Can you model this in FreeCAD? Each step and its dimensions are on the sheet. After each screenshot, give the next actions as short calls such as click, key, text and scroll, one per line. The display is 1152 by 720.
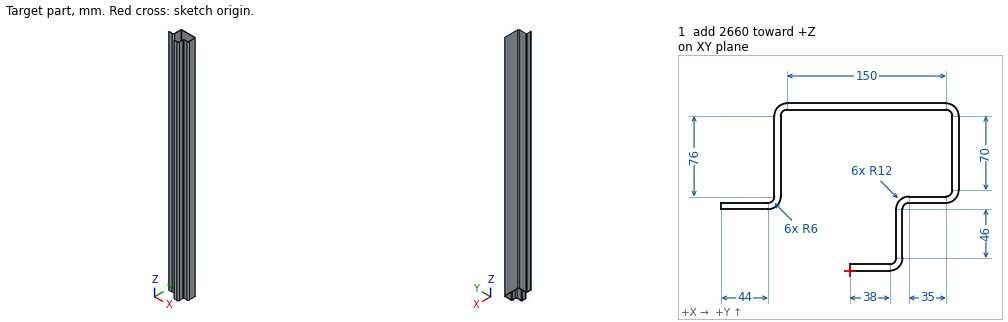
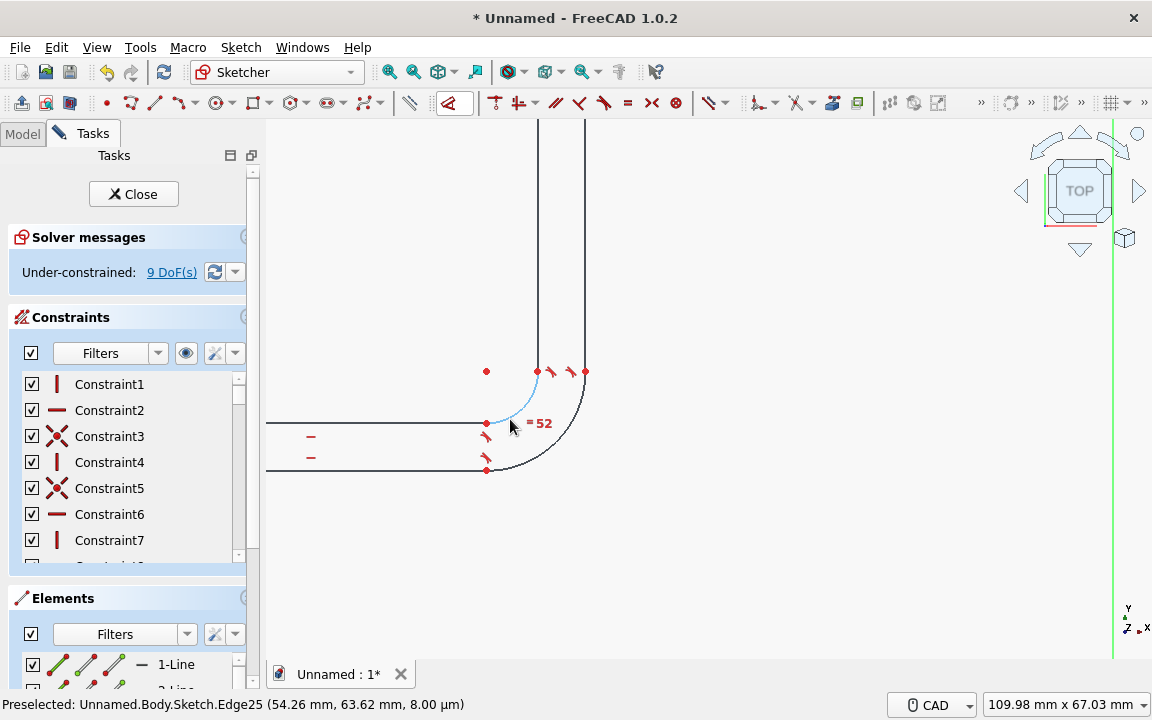
click(510, 418)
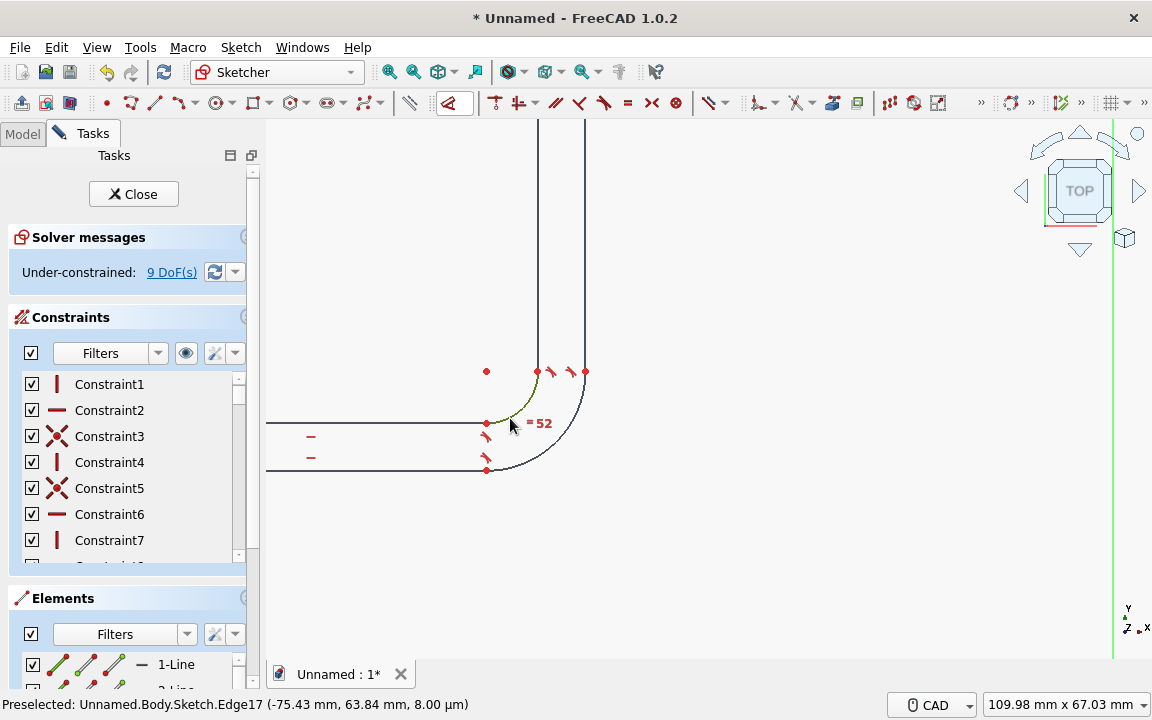
key(k)
key(r)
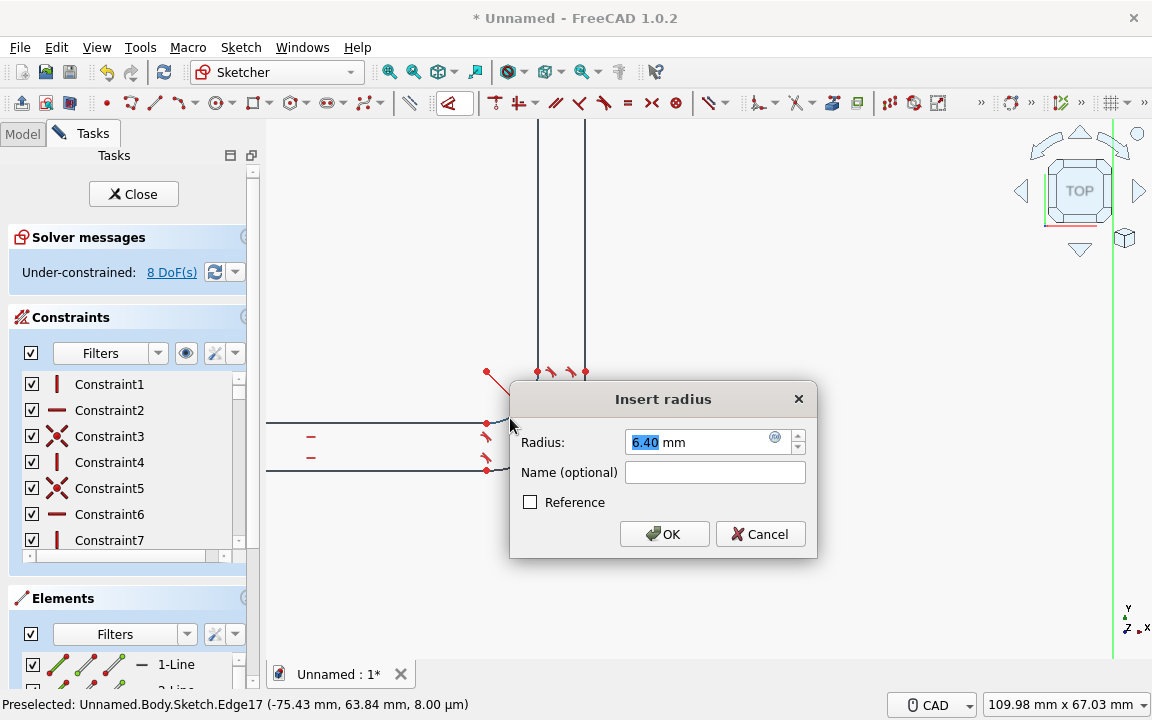
text(6)
key(Return)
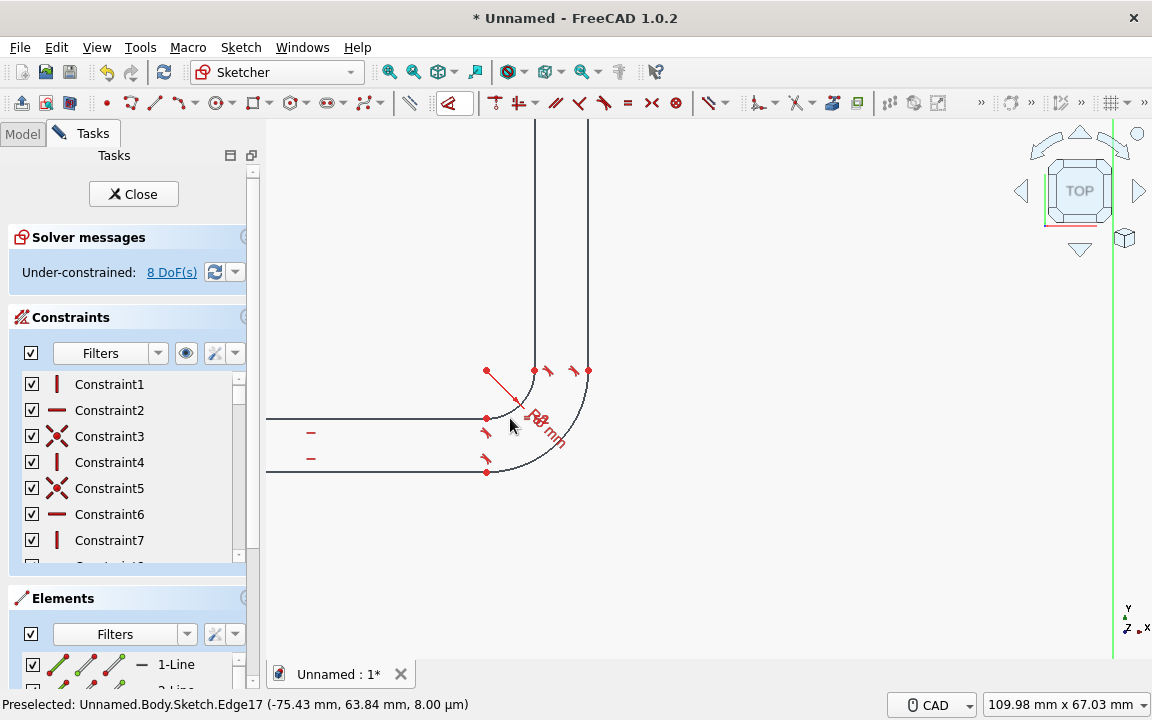
click(533, 461)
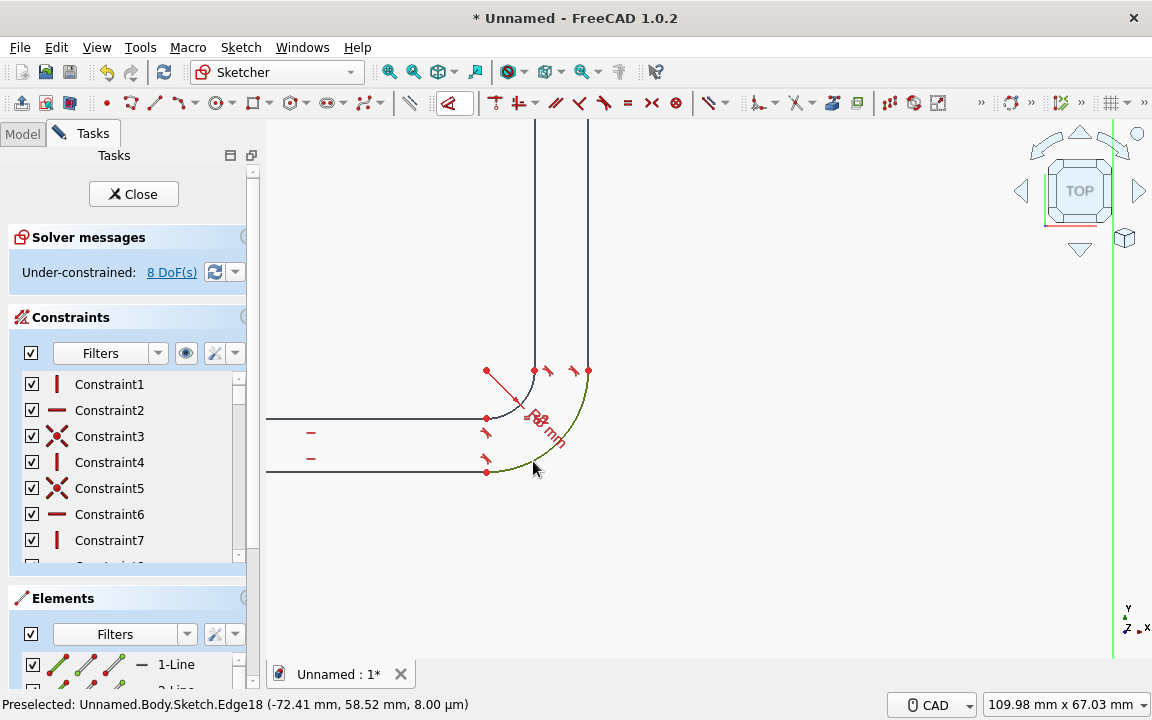
click(468, 104)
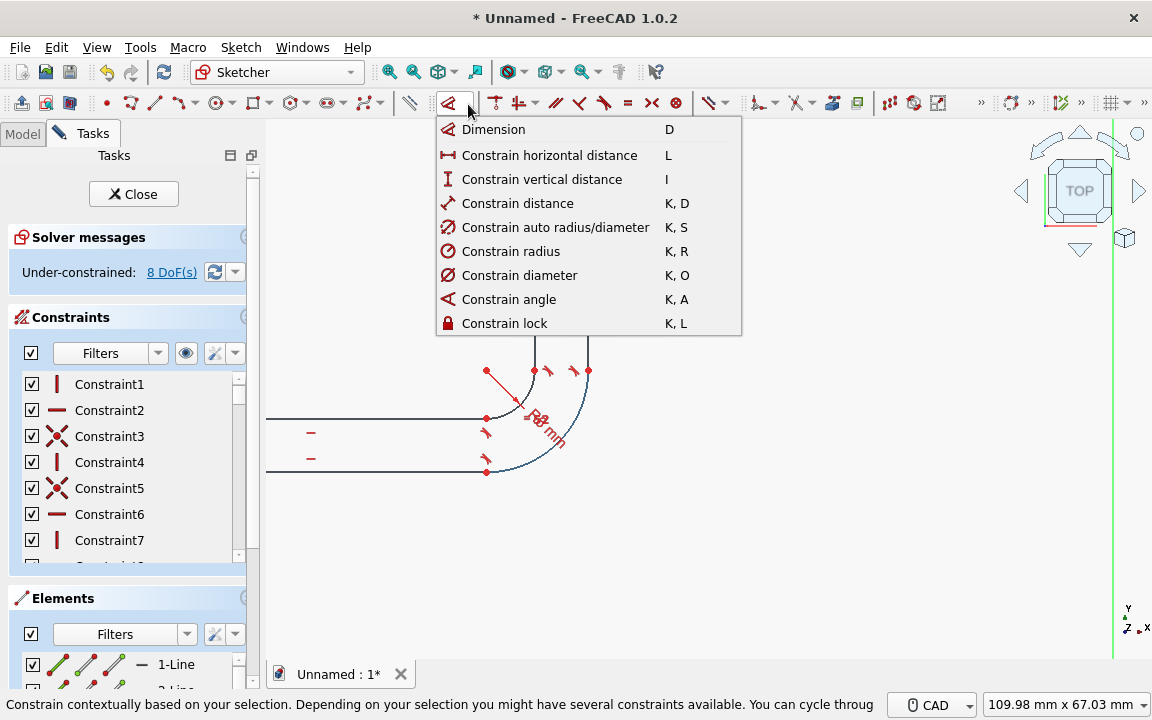
click(589, 251)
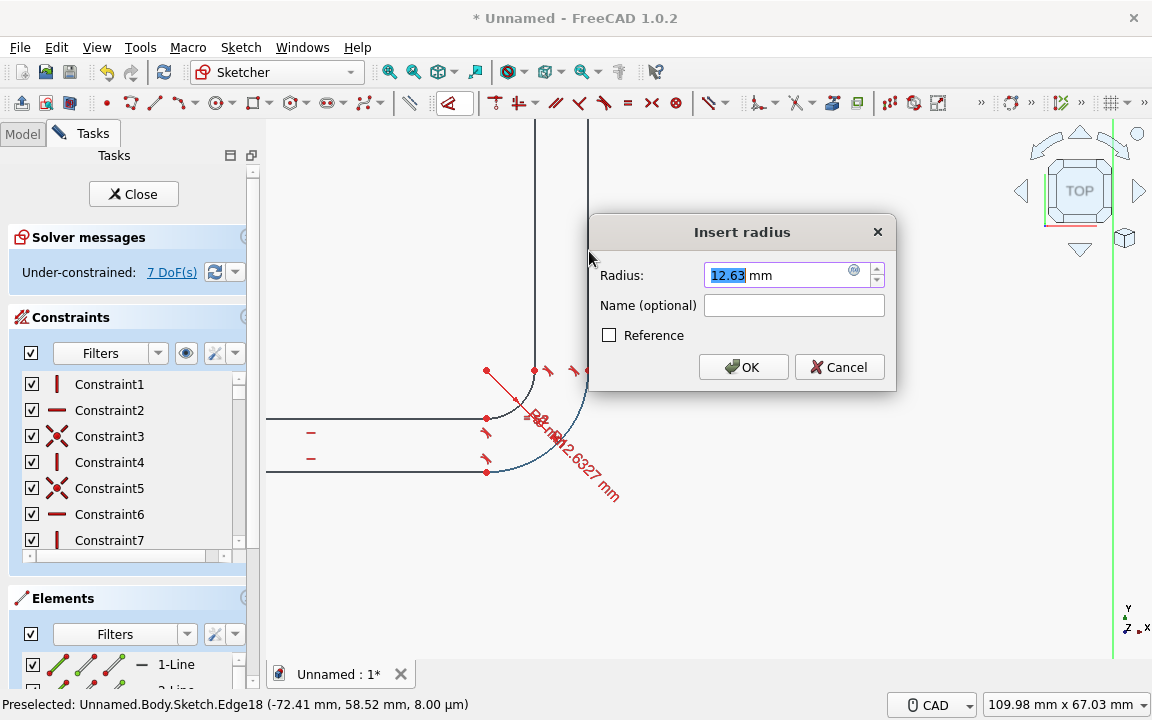
text(12)
key(Return)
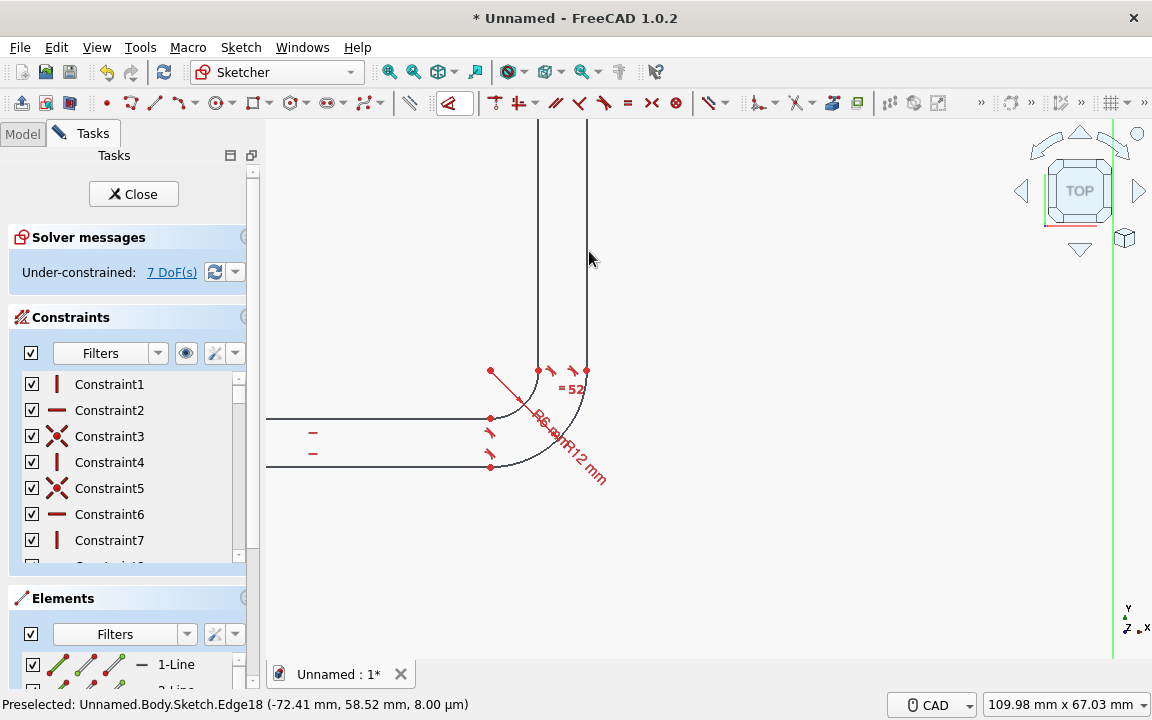
scroll(510, 419, down, 7)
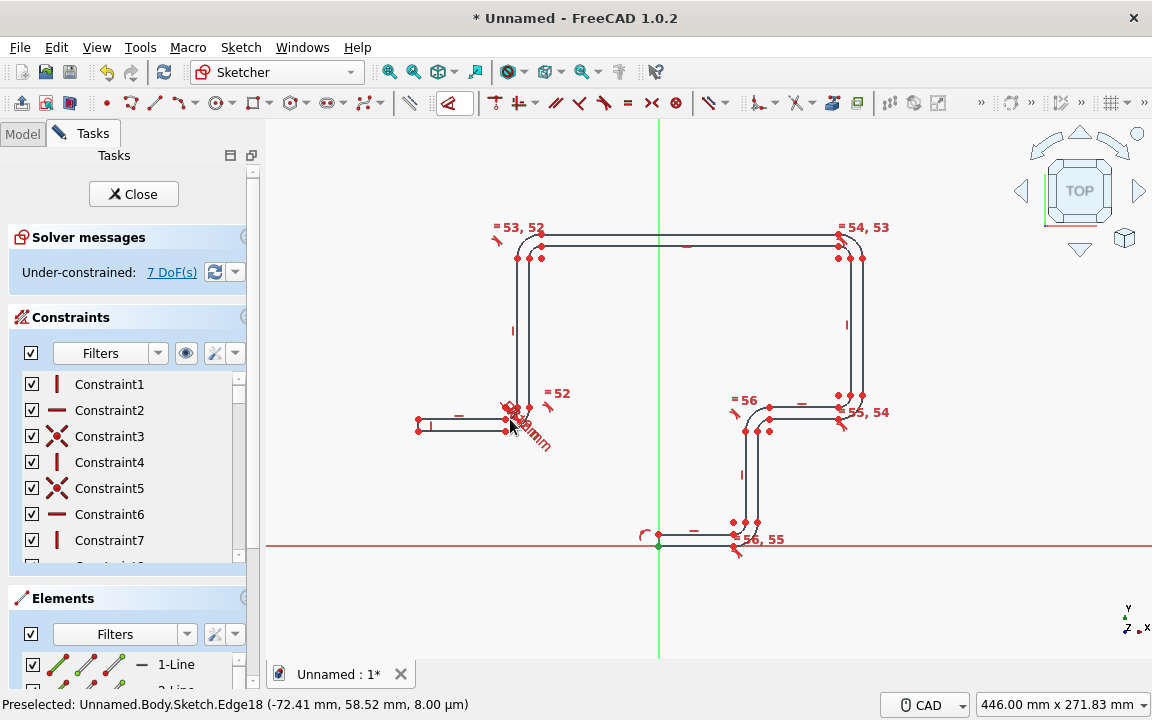
click(517, 363)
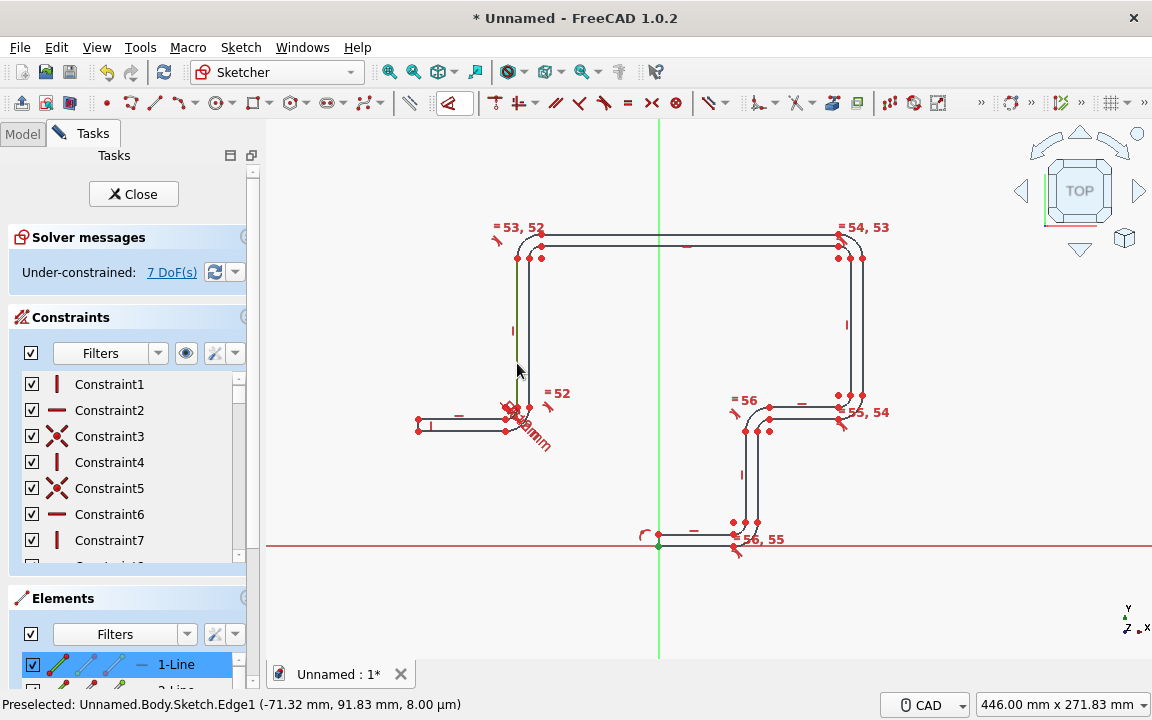
key(i)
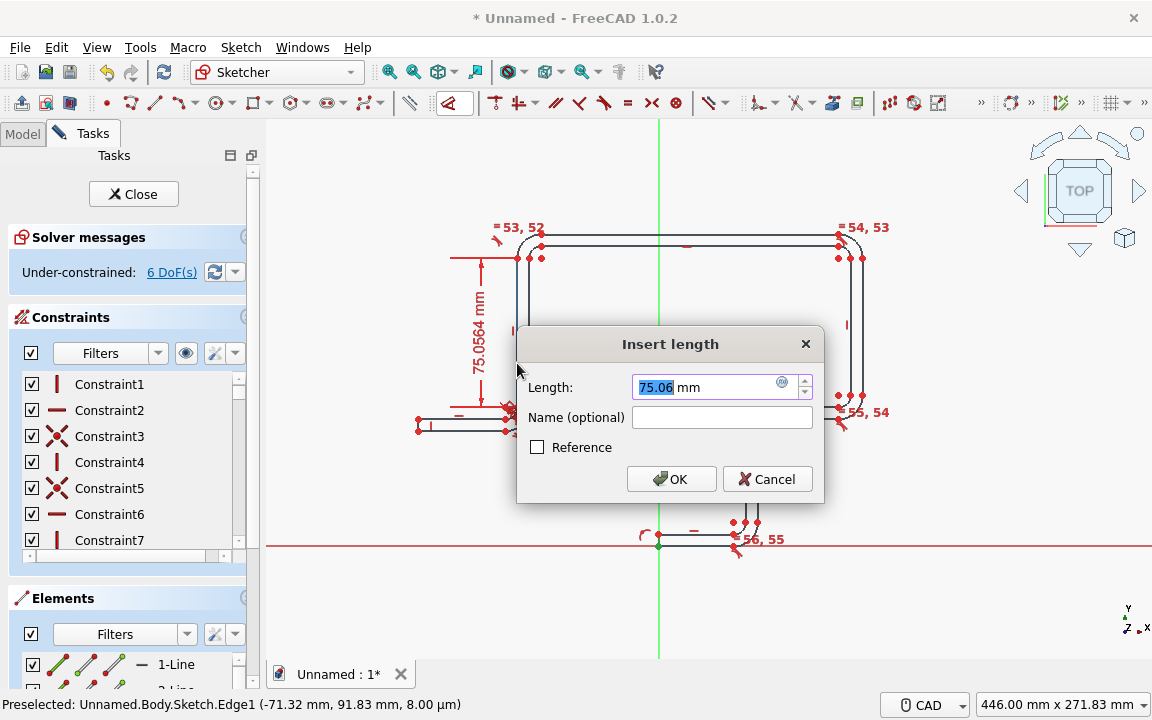
text(76)
key(Return)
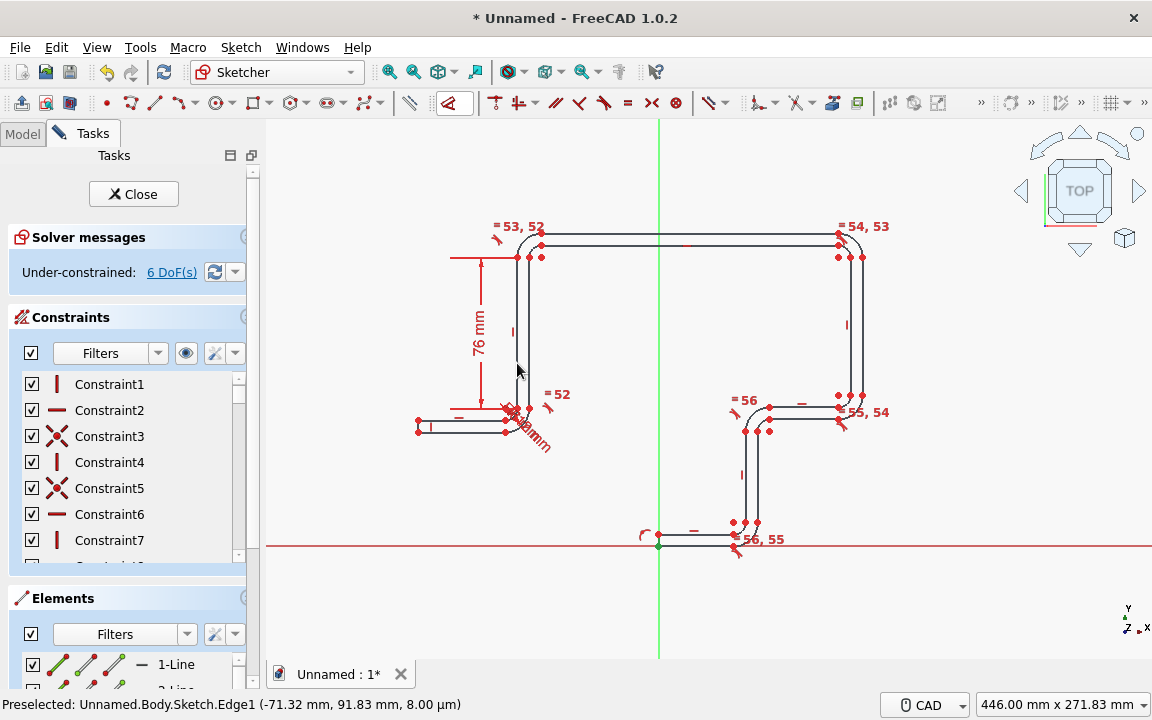
click(479, 421)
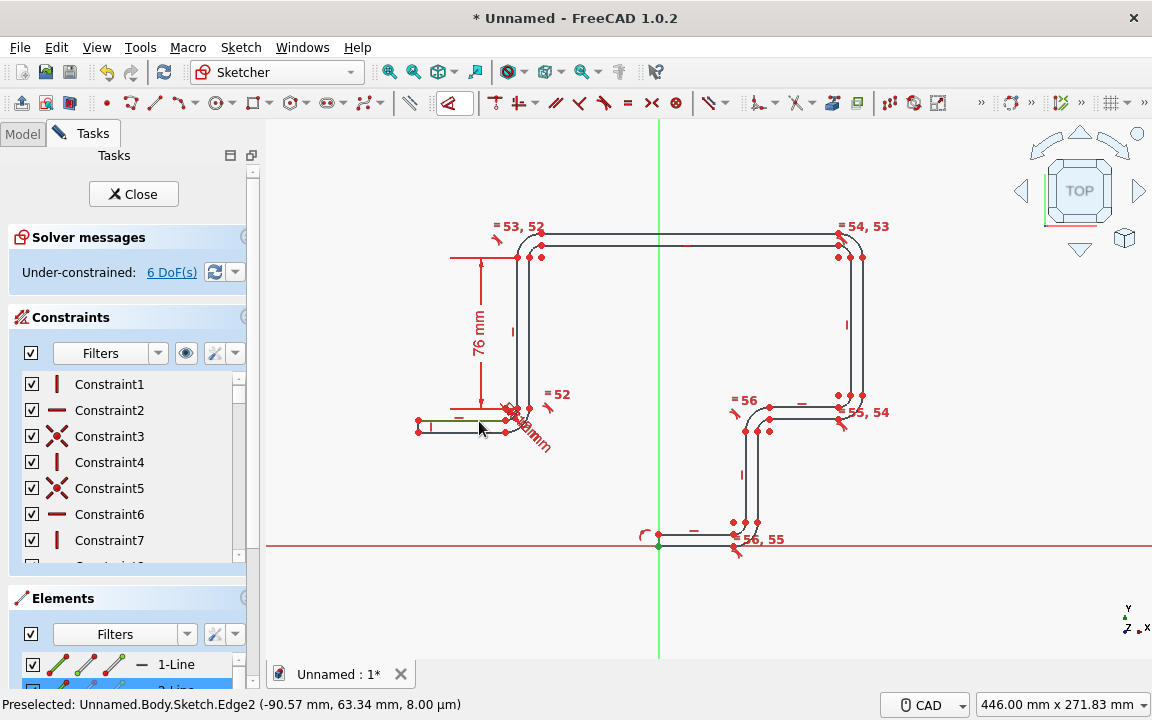
key(l)